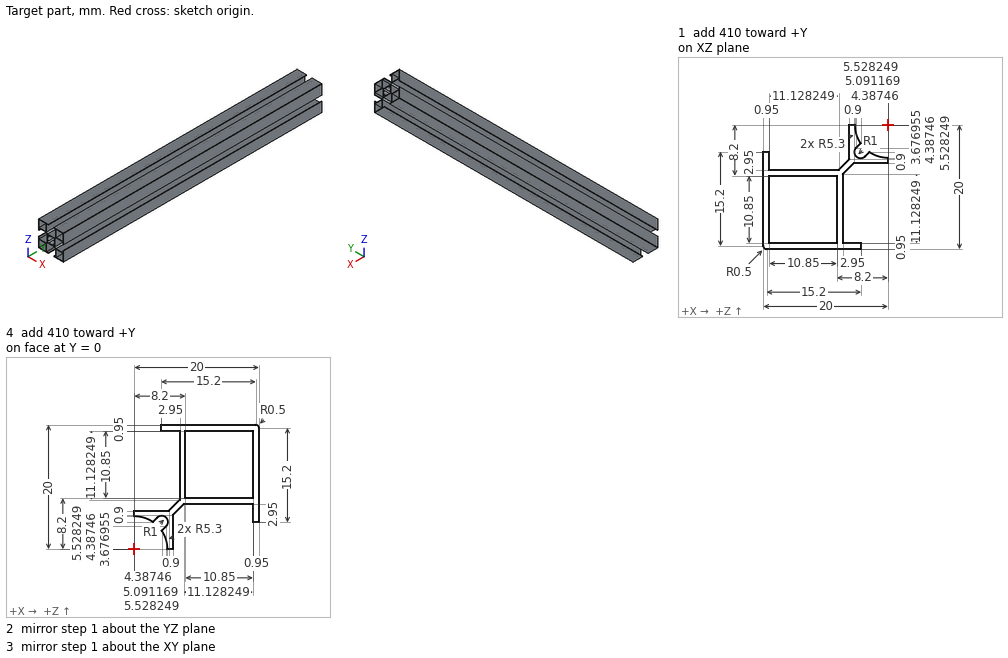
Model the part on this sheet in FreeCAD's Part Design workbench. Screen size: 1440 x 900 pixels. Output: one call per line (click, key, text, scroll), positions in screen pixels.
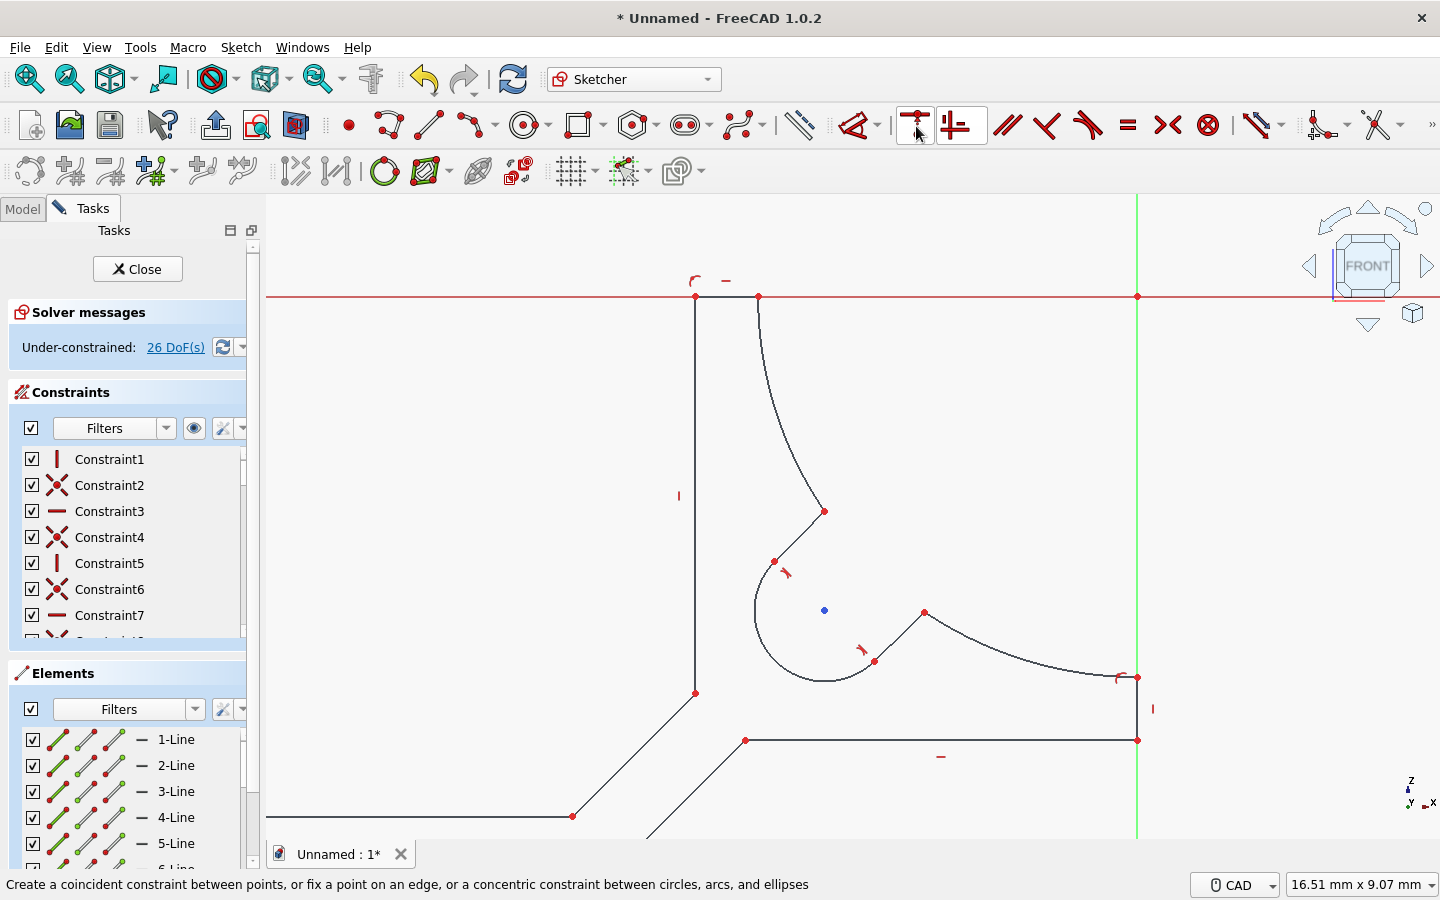
click(764, 365)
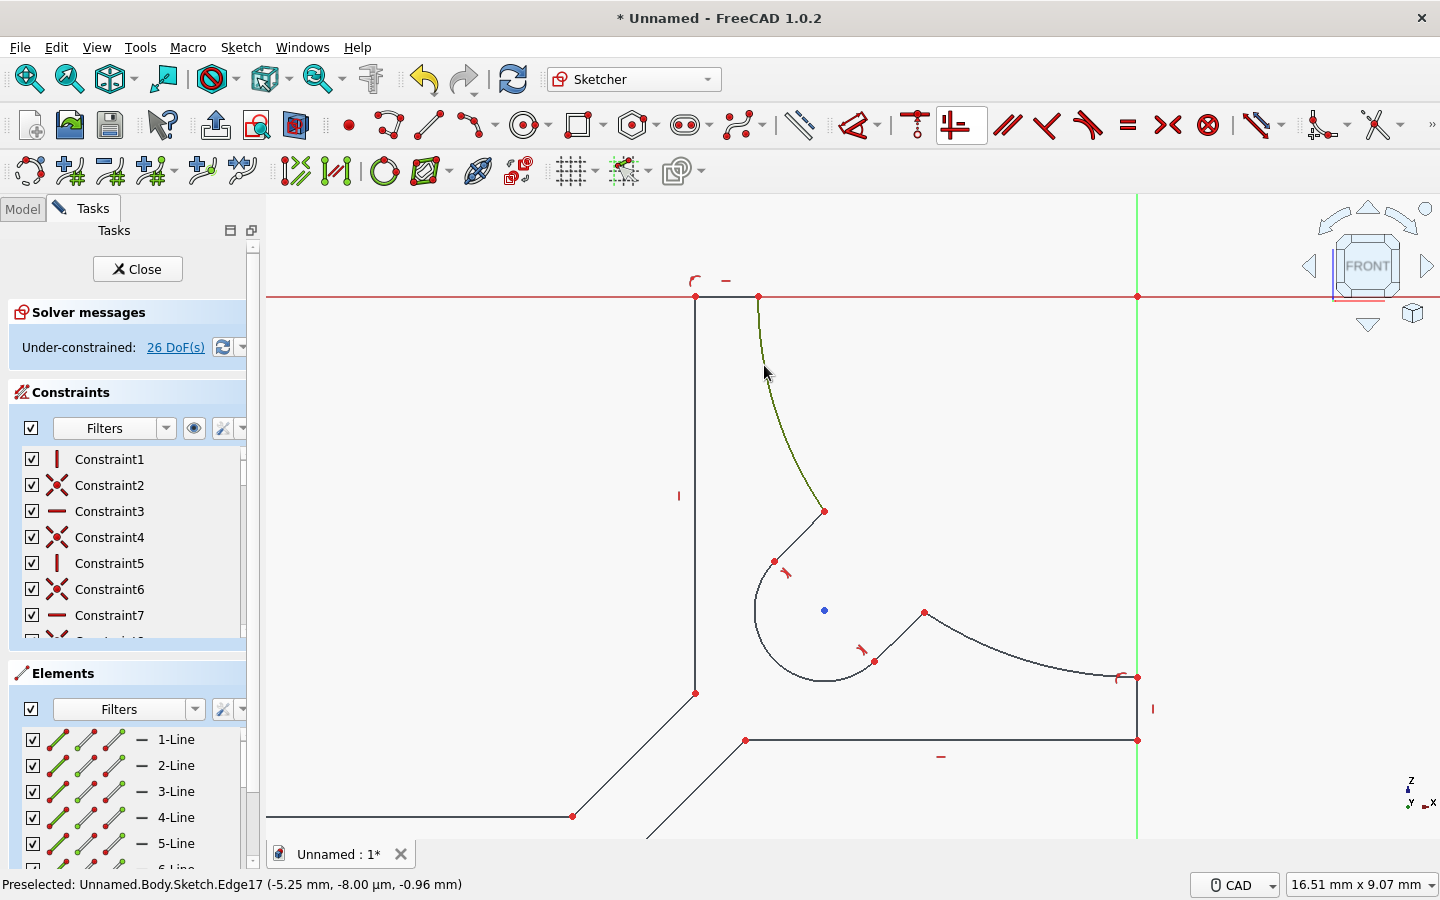
click(984, 645)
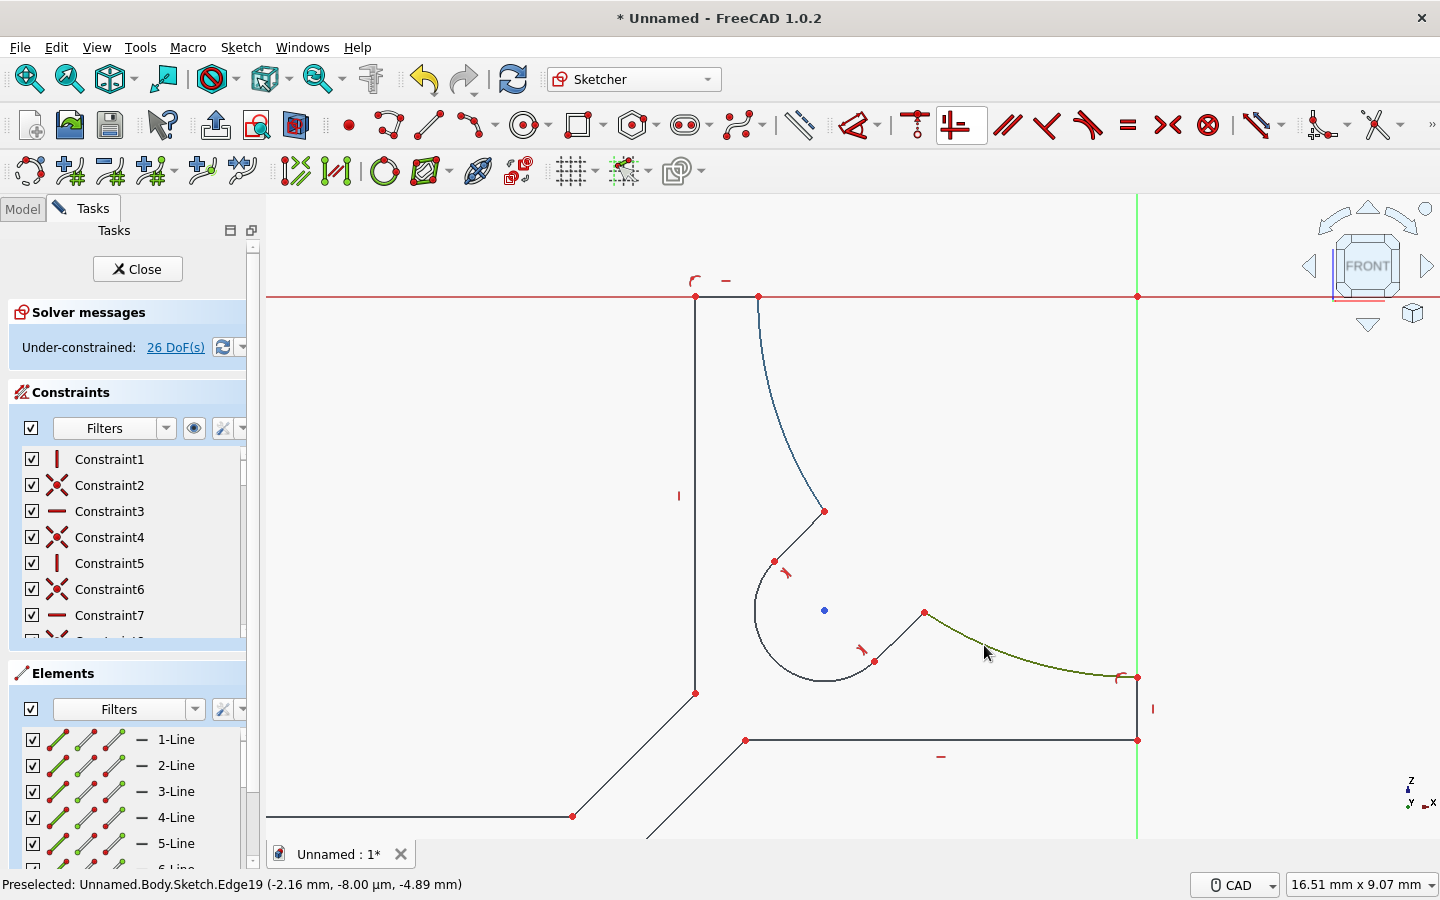
click(1128, 126)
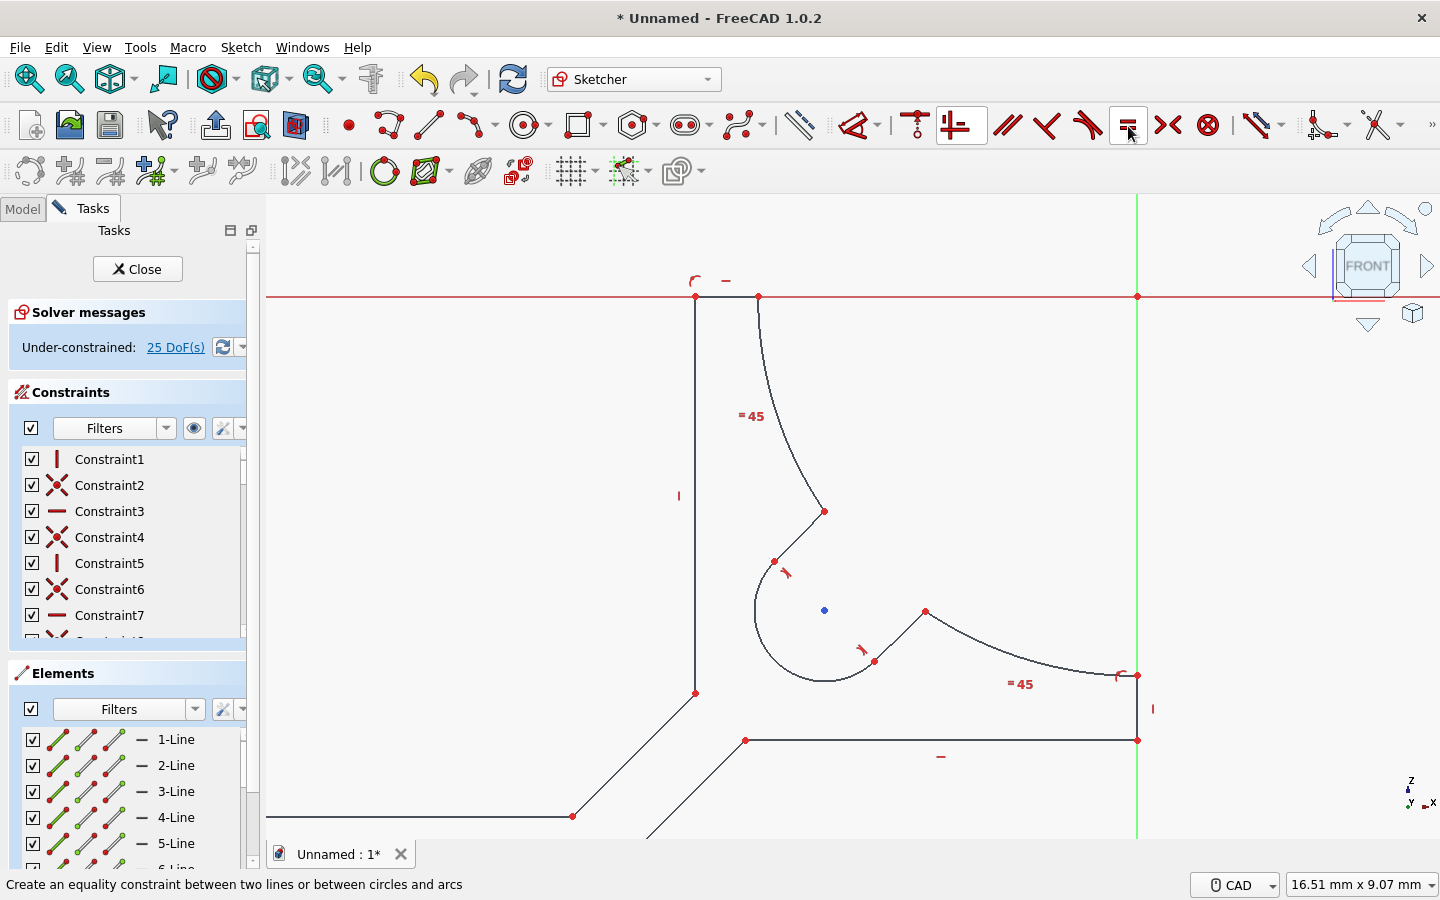
click(764, 365)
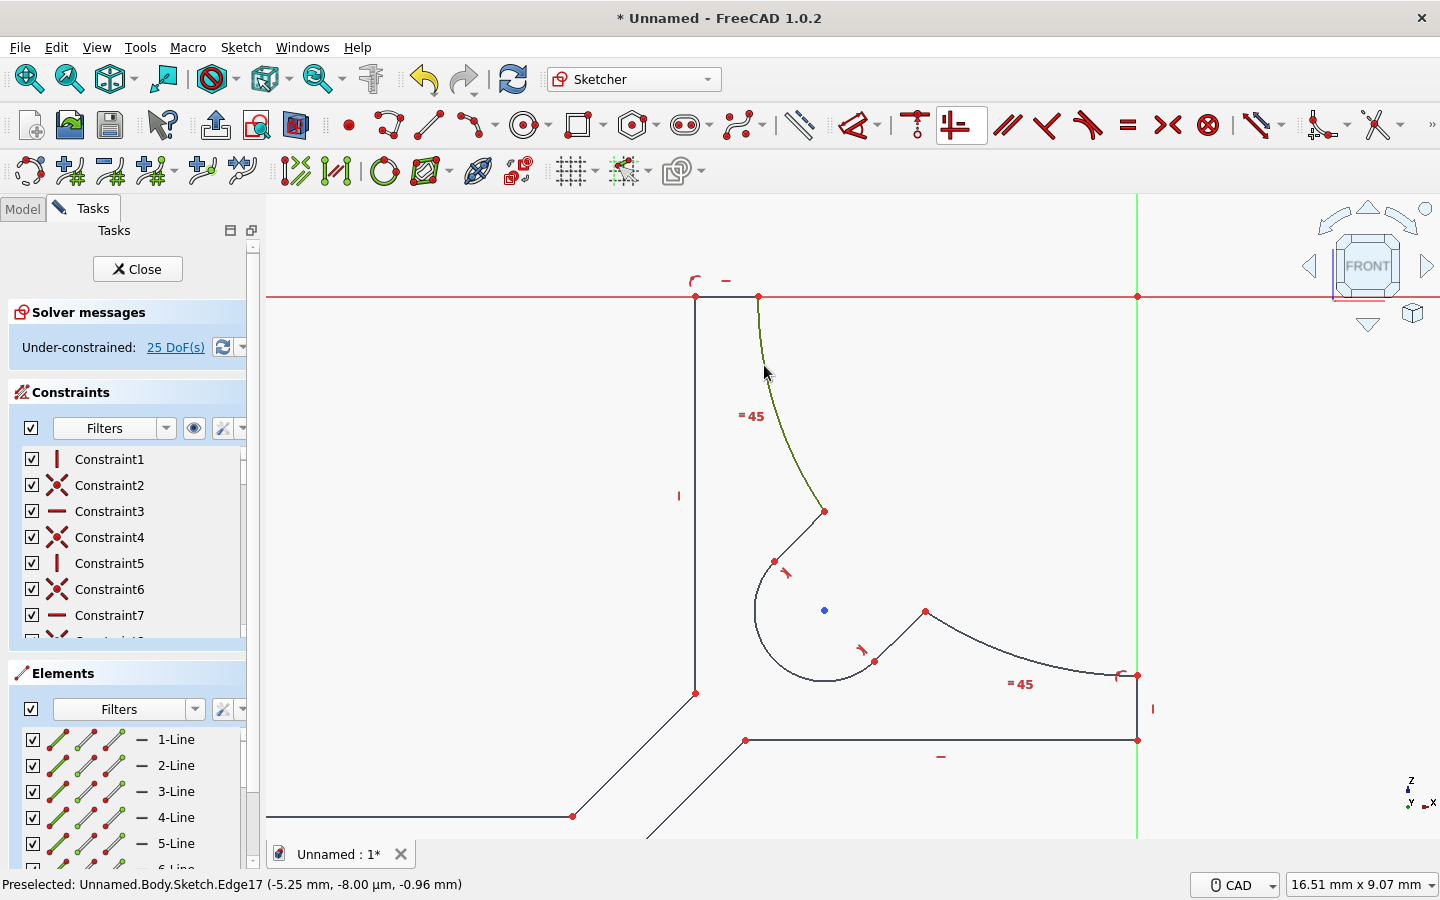
key(k)
key(r)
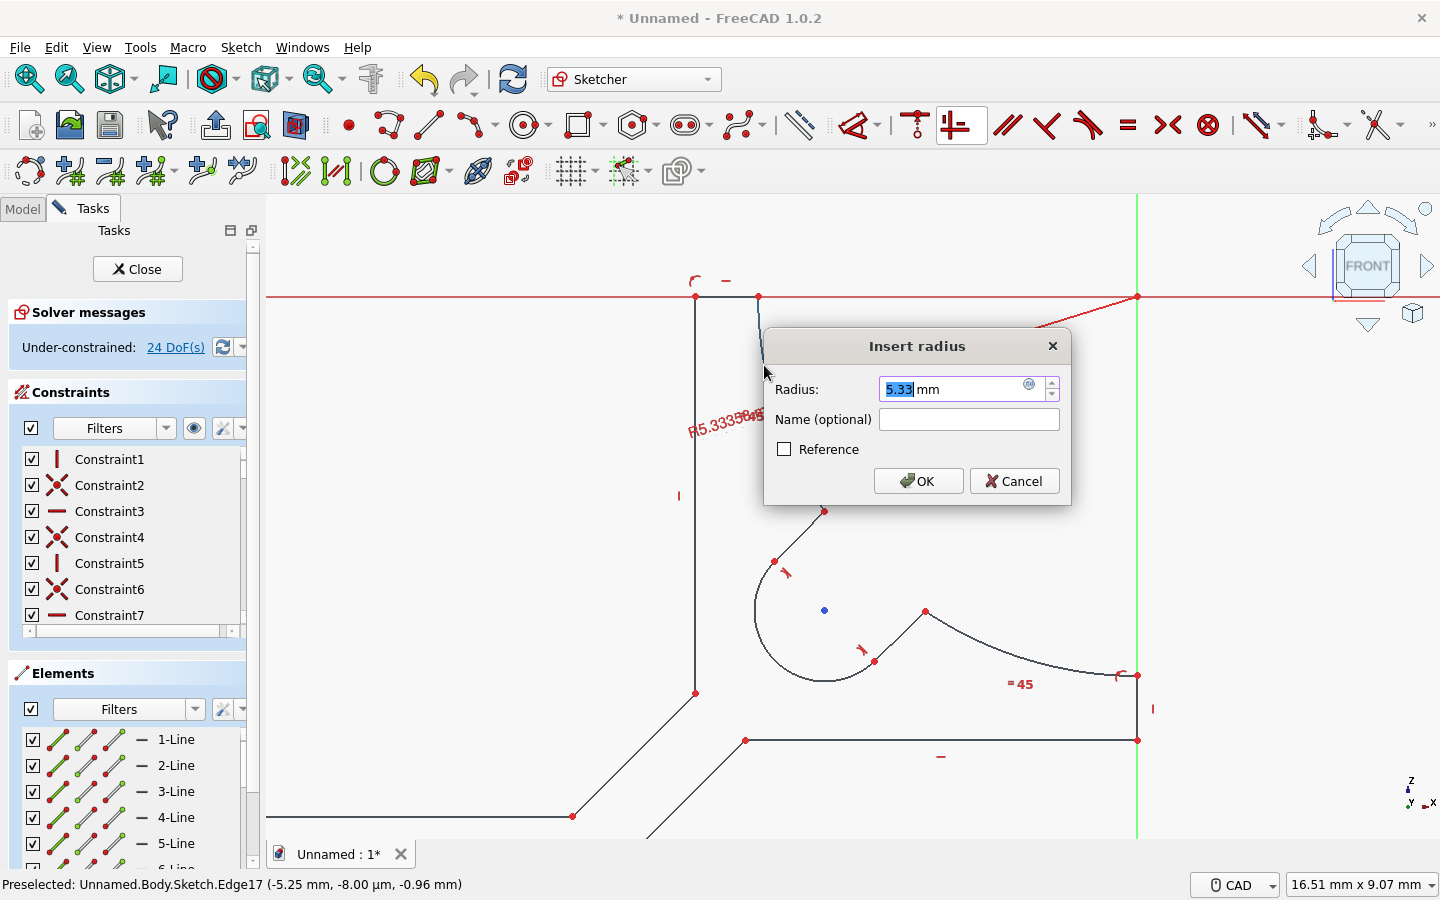
text(5.3)
key(Return)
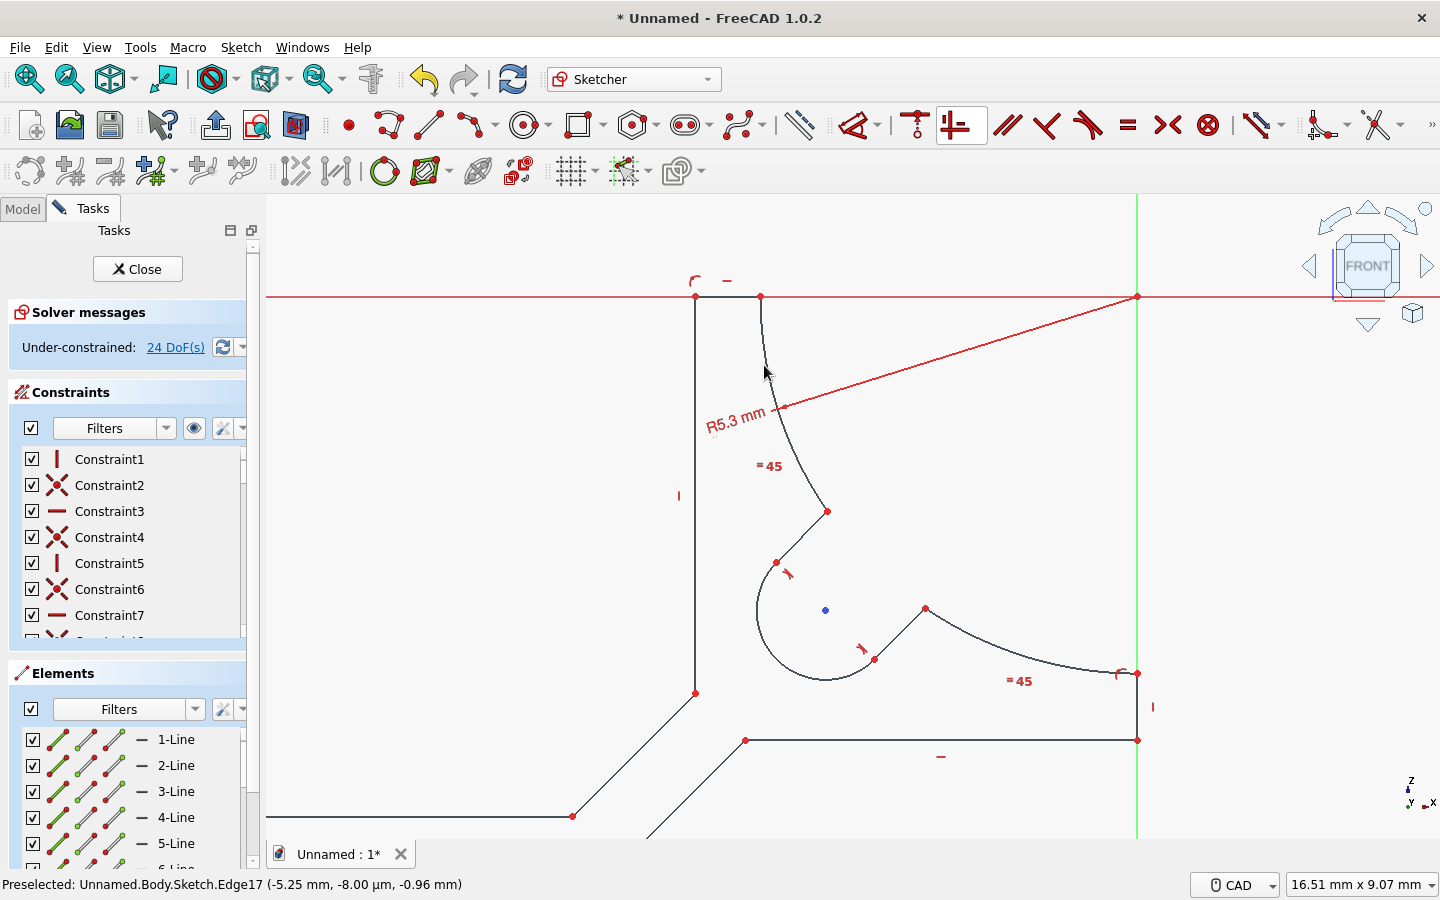
click(758, 622)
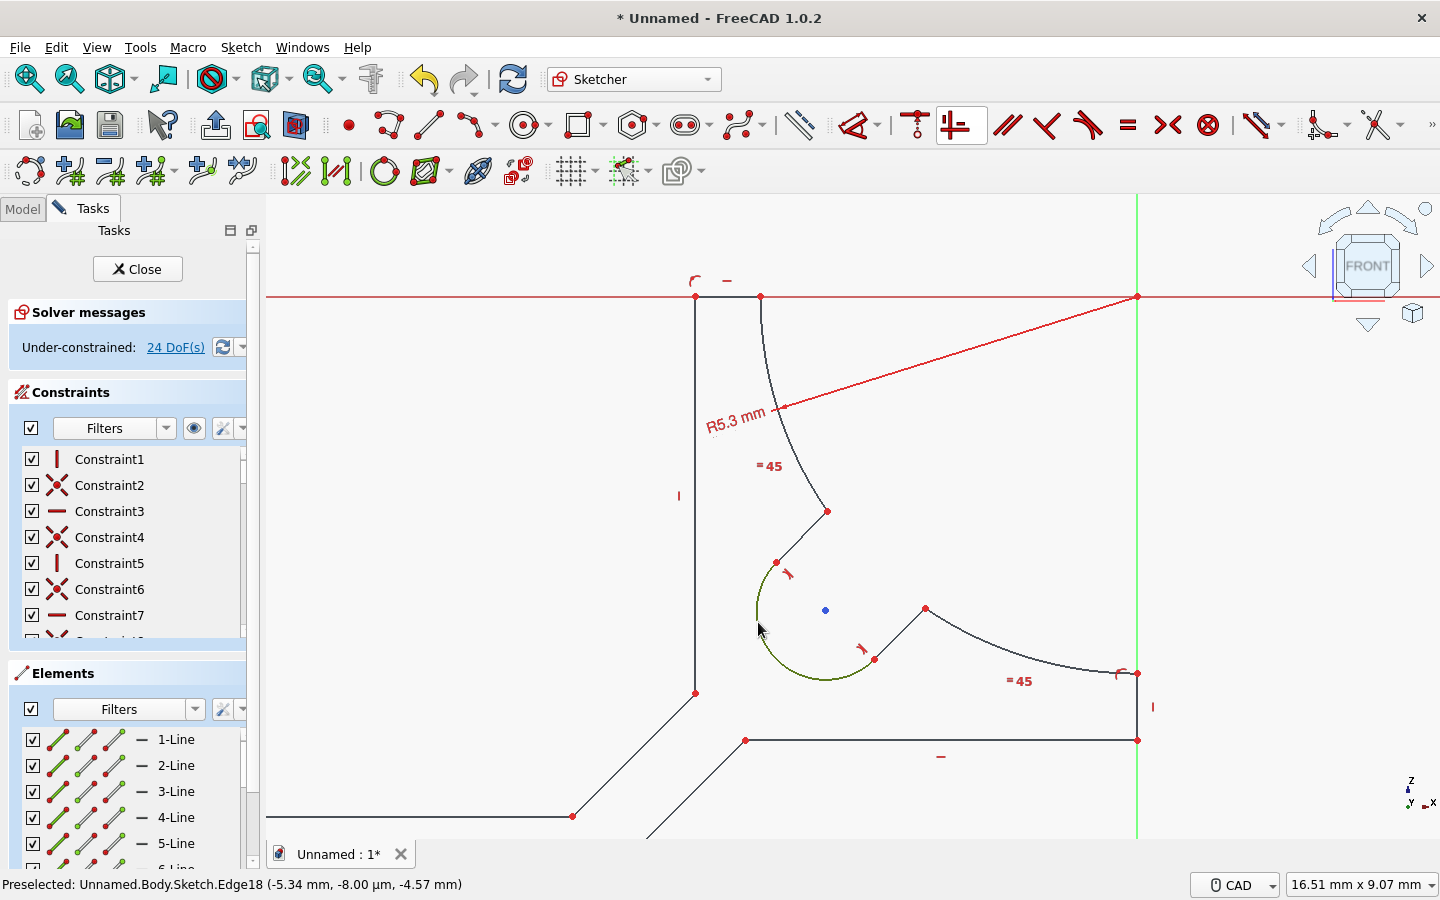
key(k)
key(r)